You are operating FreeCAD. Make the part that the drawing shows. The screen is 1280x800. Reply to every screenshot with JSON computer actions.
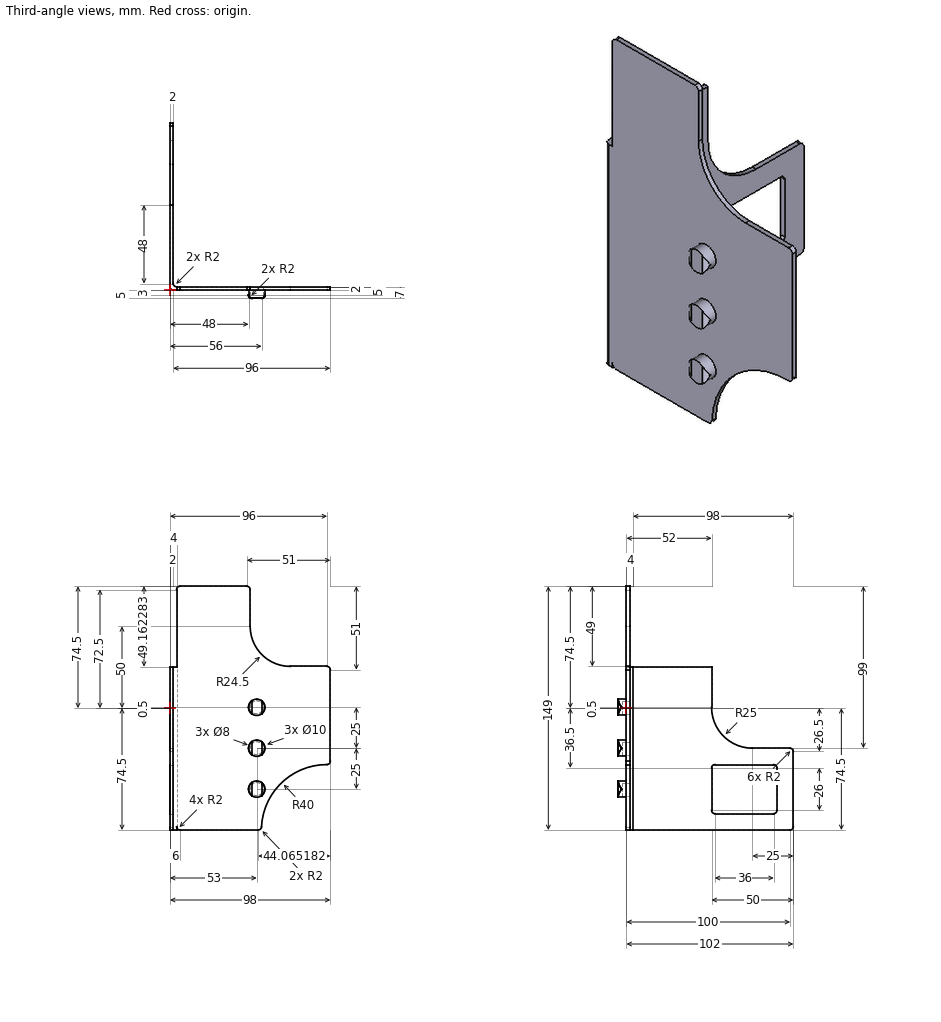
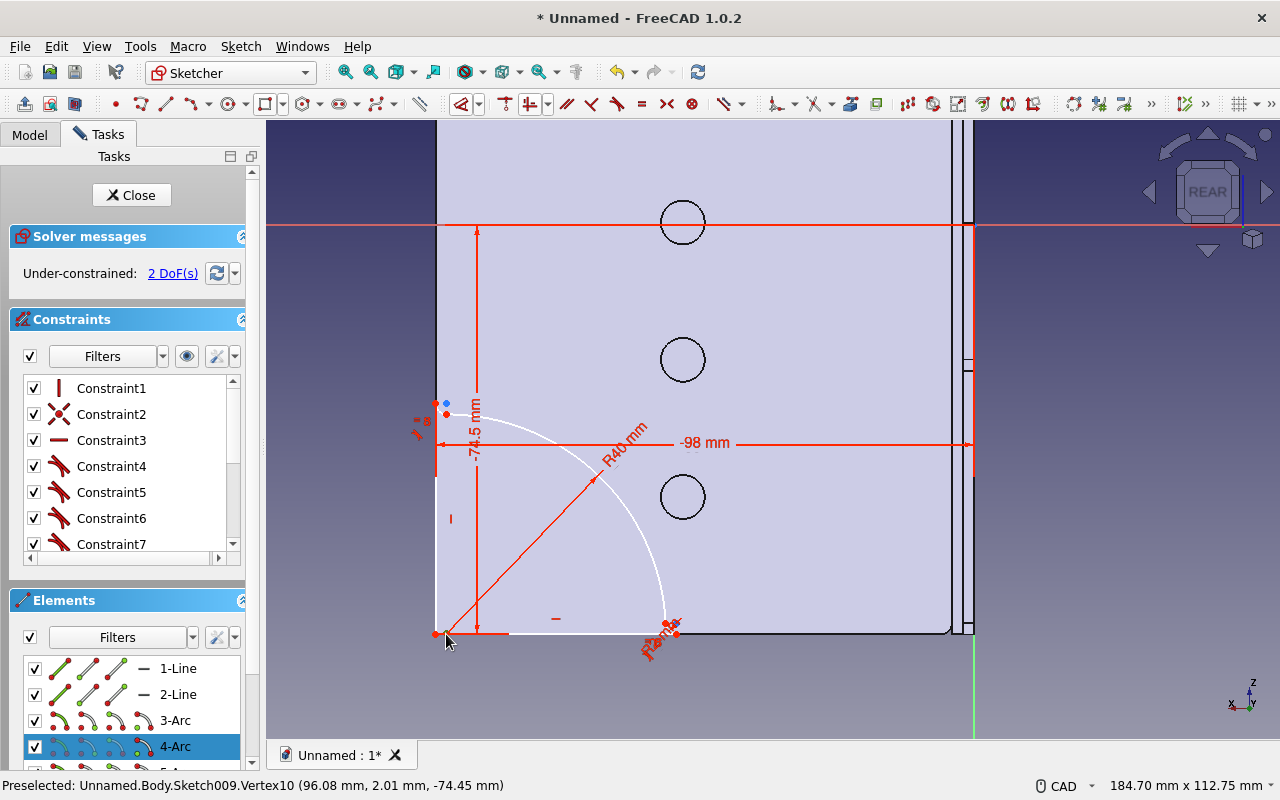
{"action": "left_click", "coordinate": [478, 104]}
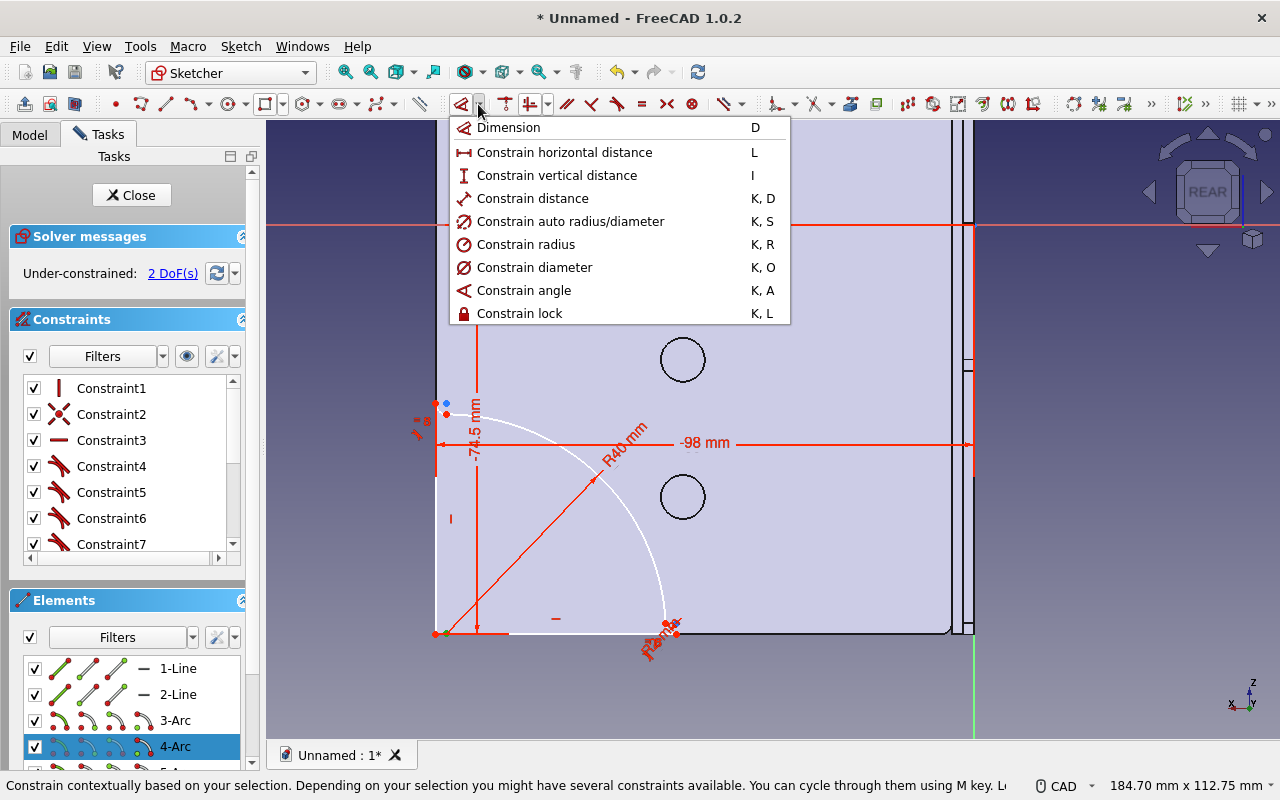
{"action": "left_click", "coordinate": [620, 176]}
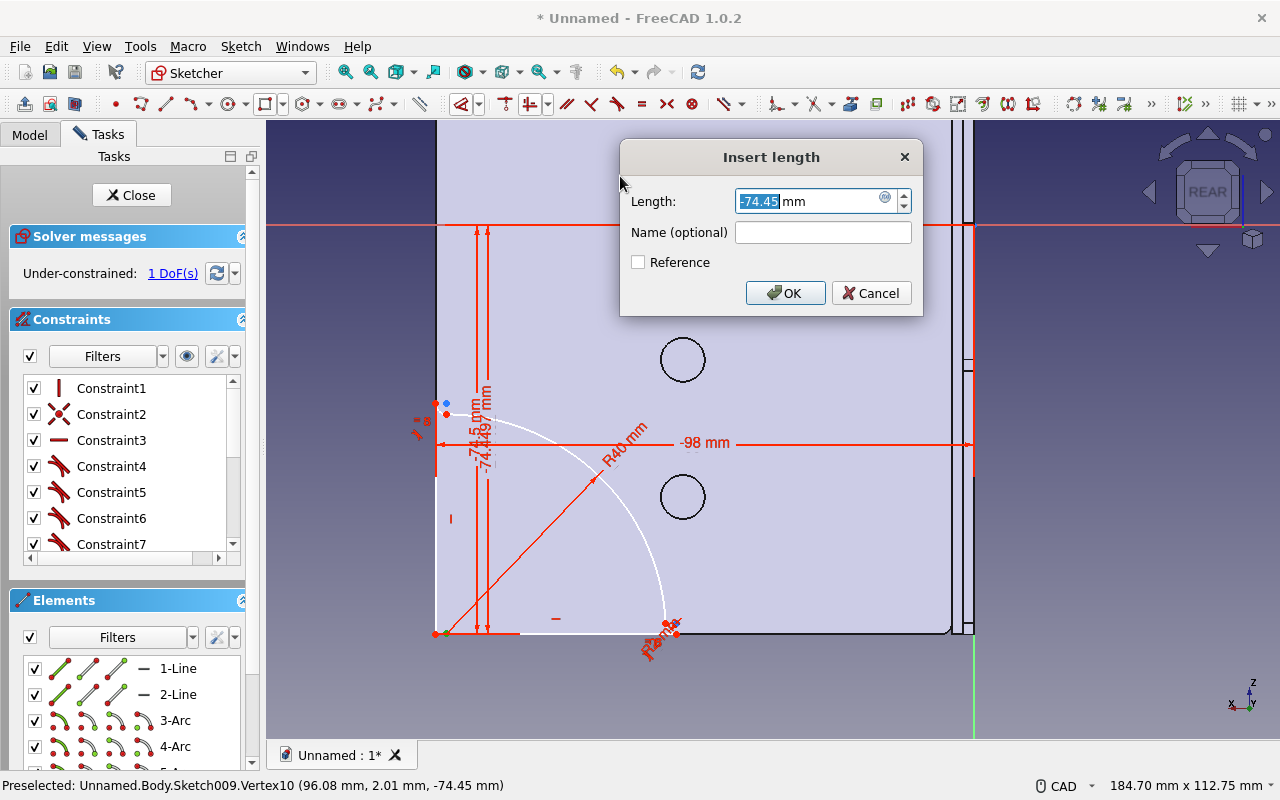
{"action": "type", "text": "-74.5"}
{"action": "key", "text": "Return"}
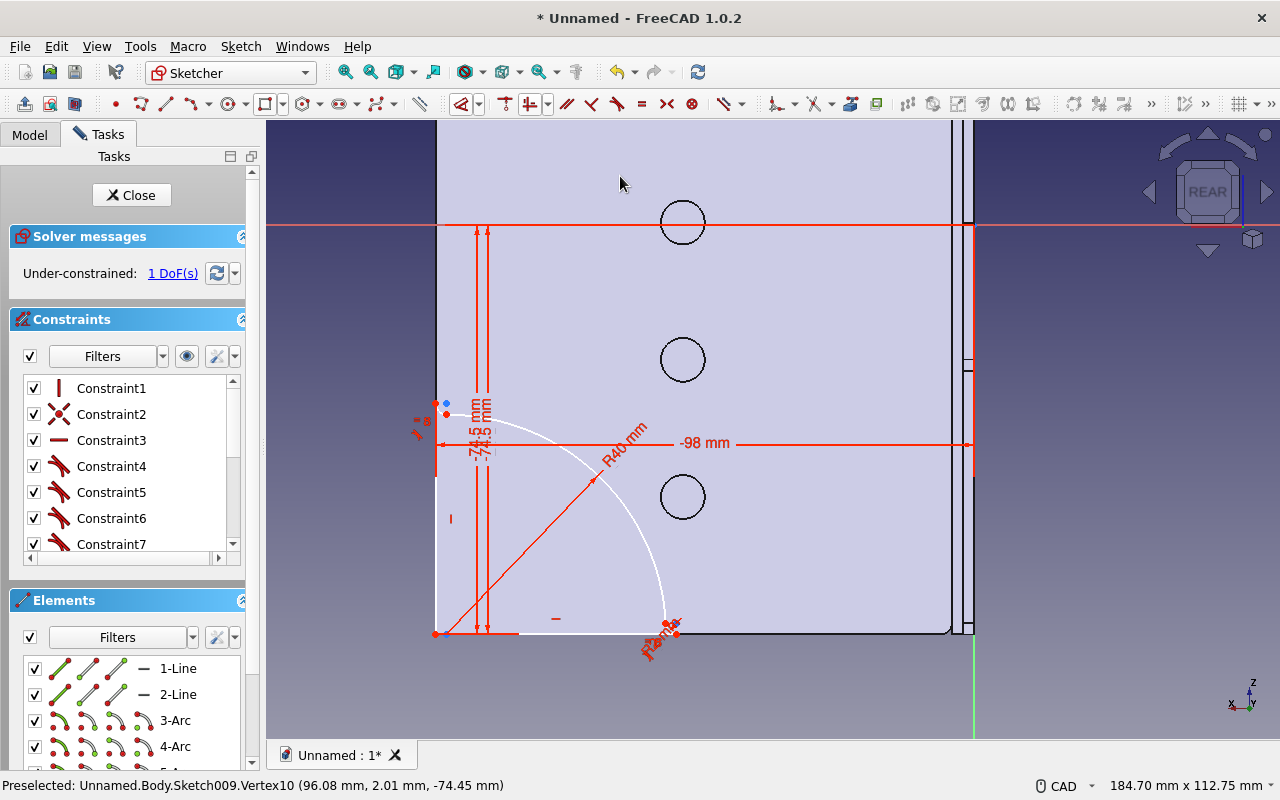
{"action": "left_click", "coordinate": [508, 634]}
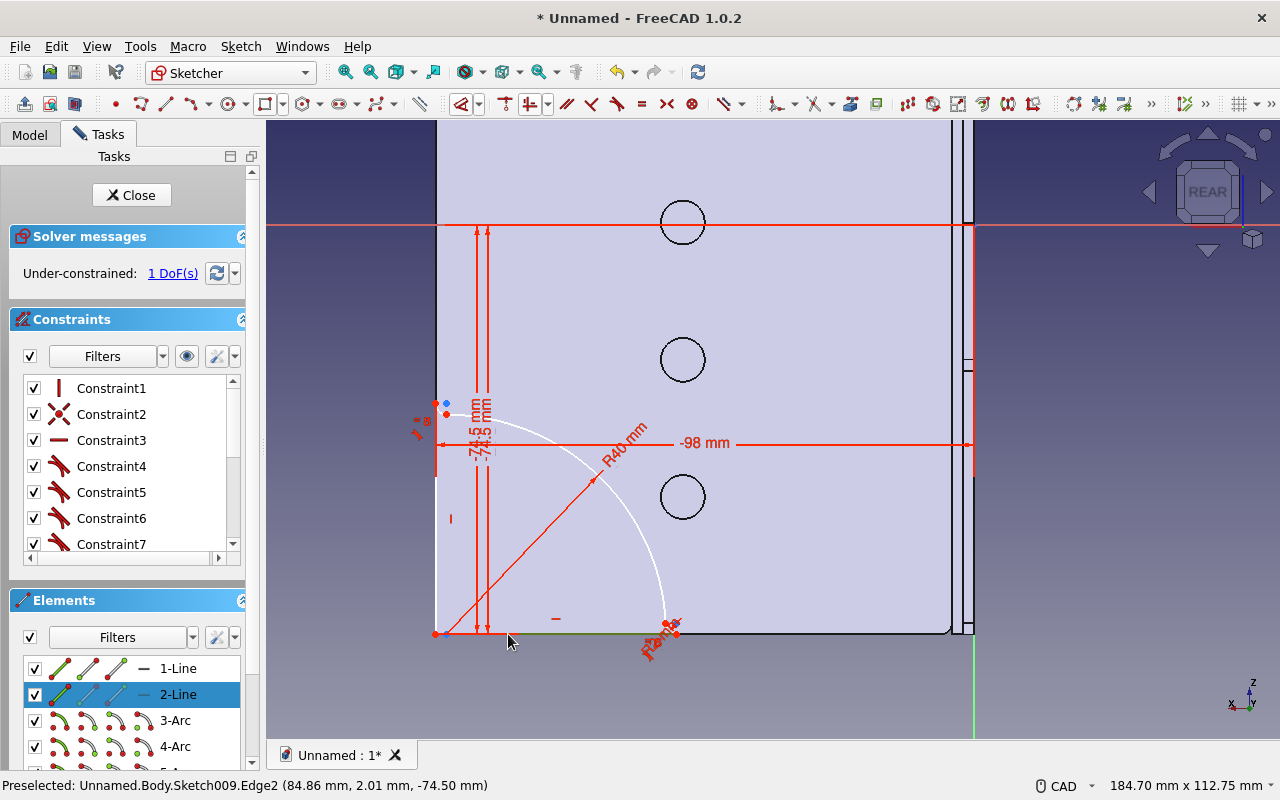
{"action": "key", "text": "l"}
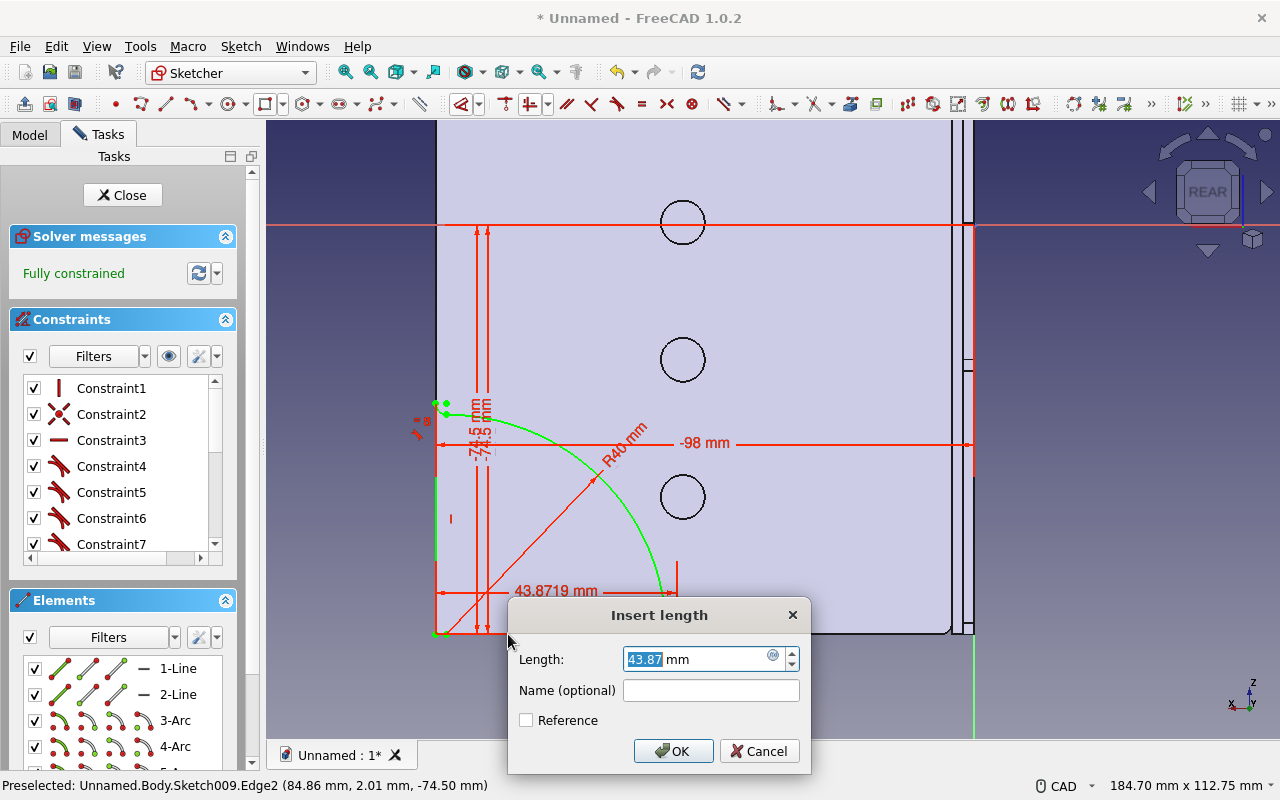
{"action": "type", "text": "44.065182"}
{"action": "key", "text": "Return"}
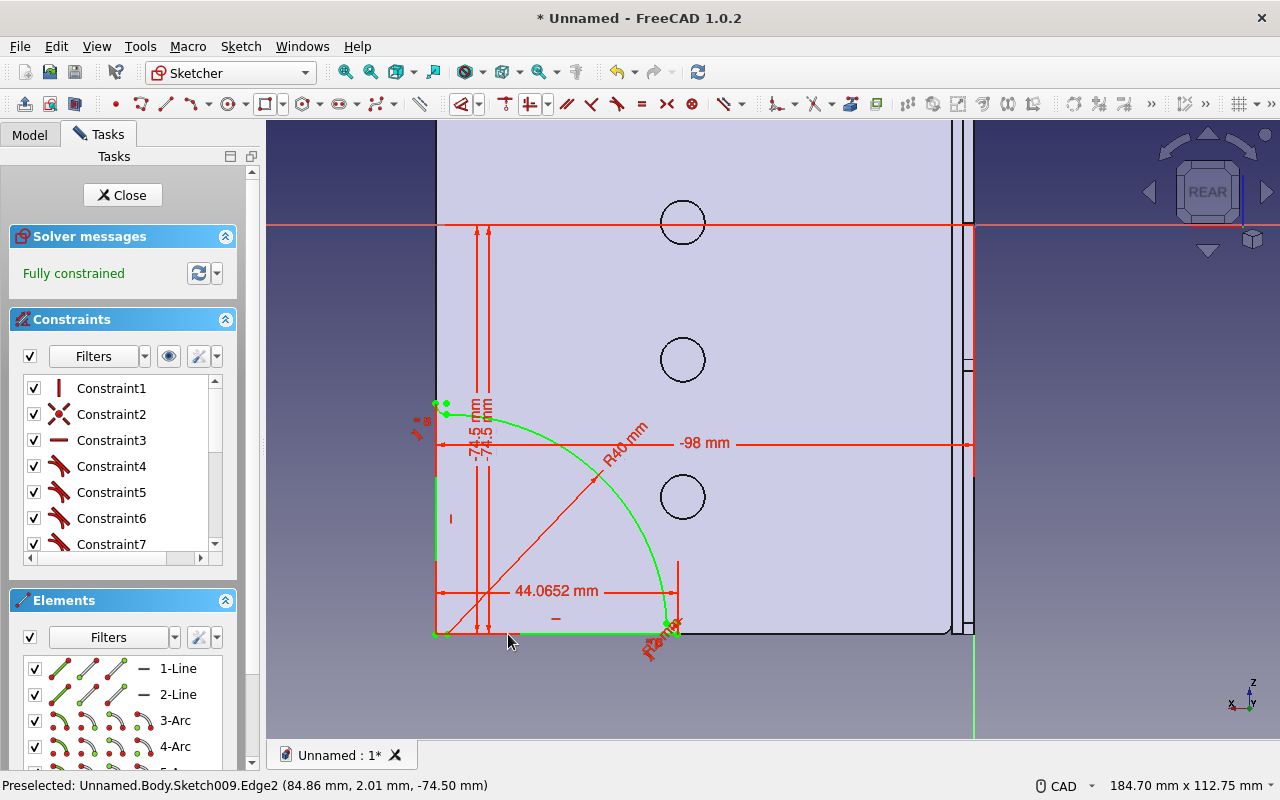
{"action": "left_click", "coordinate": [123, 195]}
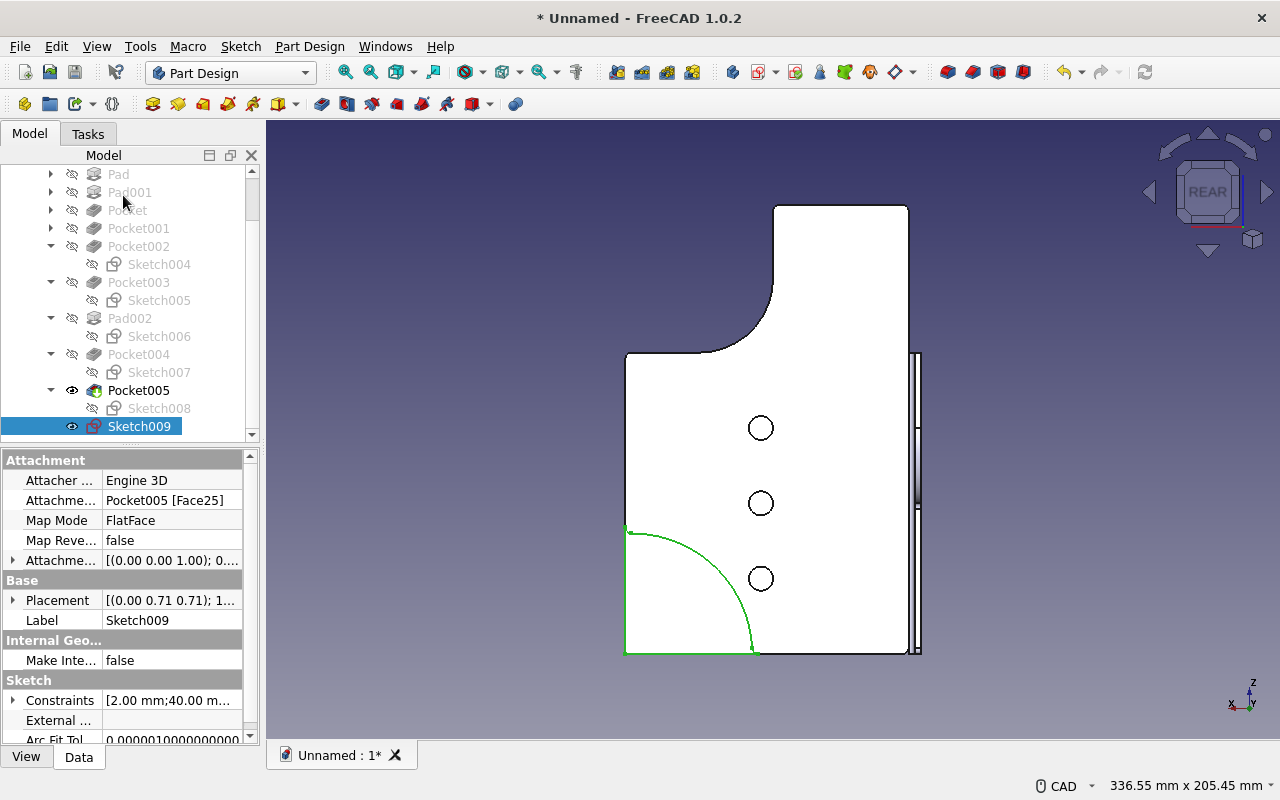
{"action": "left_click", "coordinate": [322, 104]}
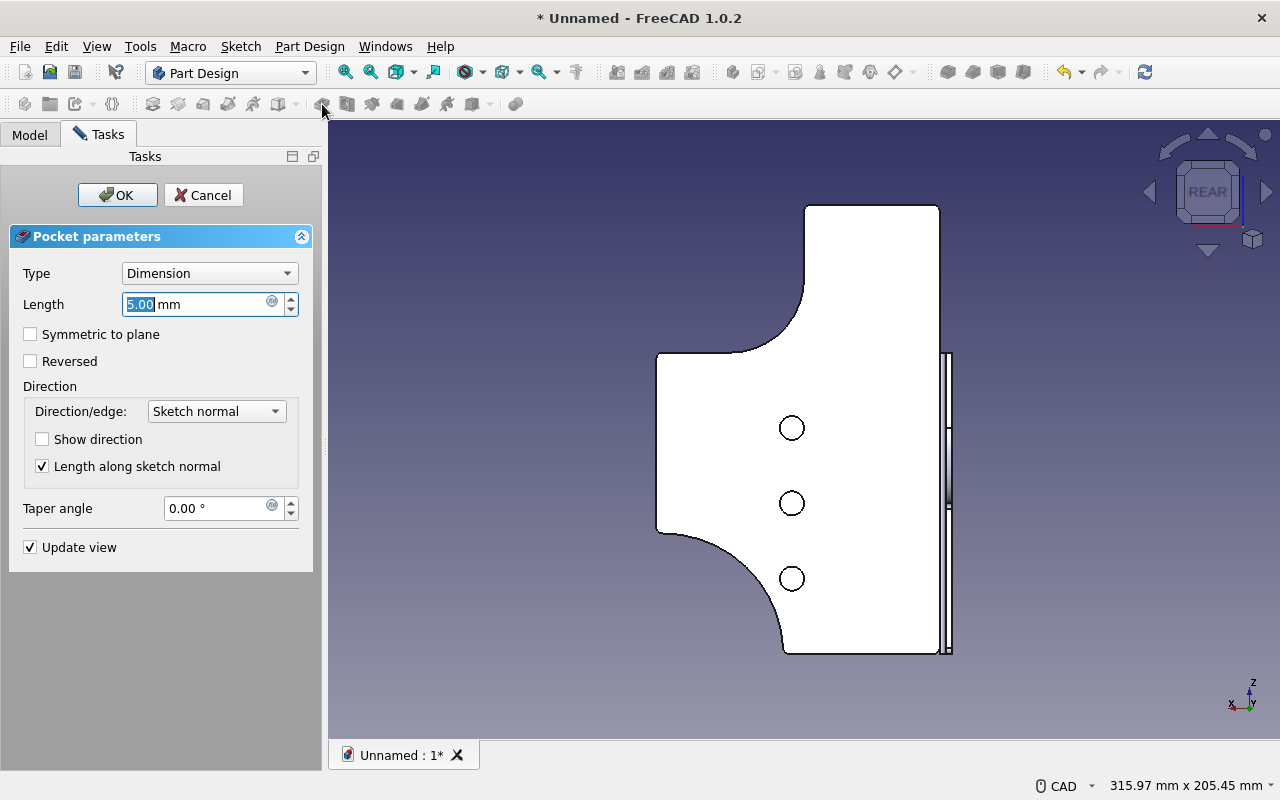
{"action": "type", "text": "5"}
{"action": "key", "text": "Tab"}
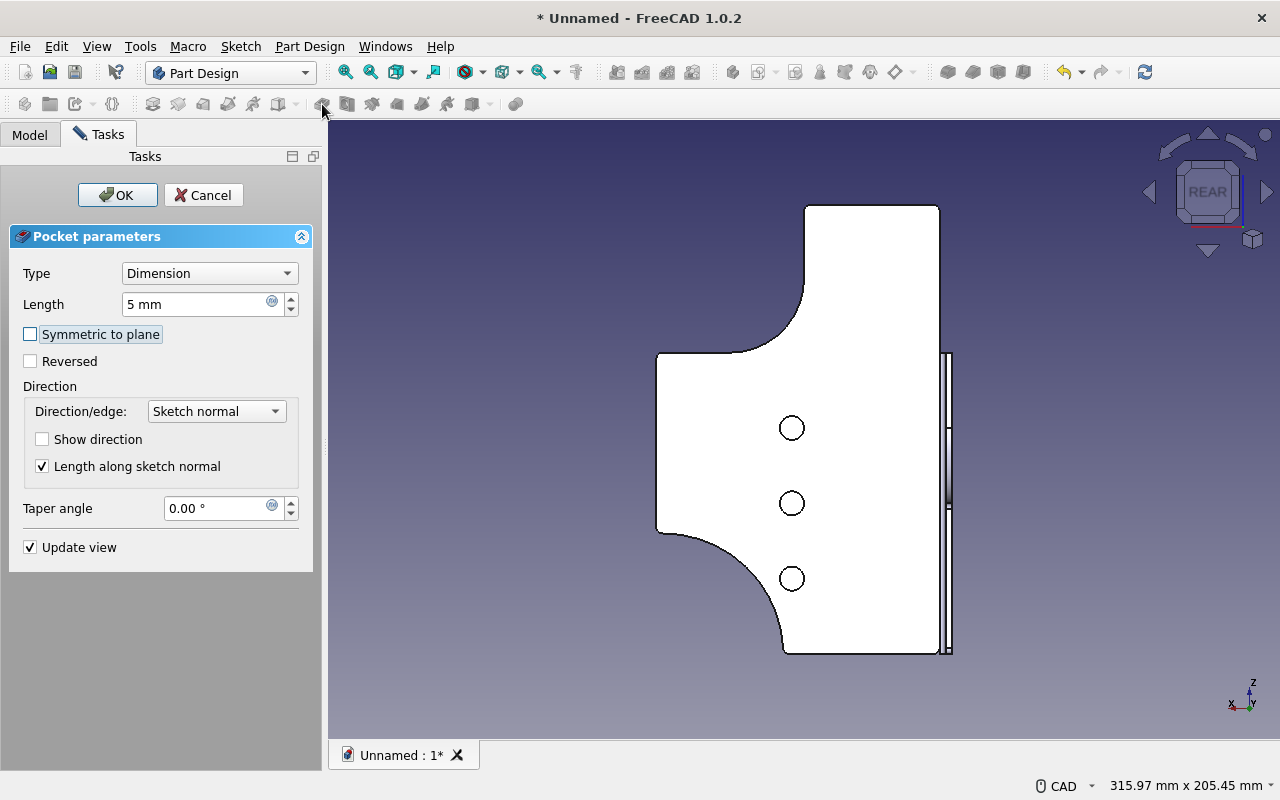
{"action": "left_click", "coordinate": [118, 195]}